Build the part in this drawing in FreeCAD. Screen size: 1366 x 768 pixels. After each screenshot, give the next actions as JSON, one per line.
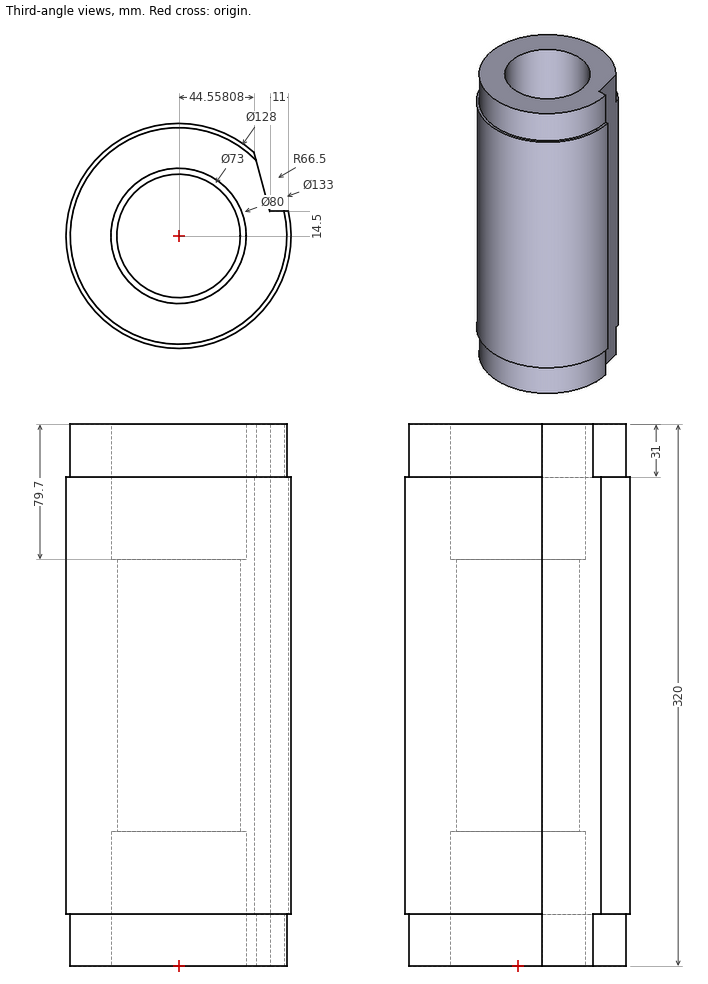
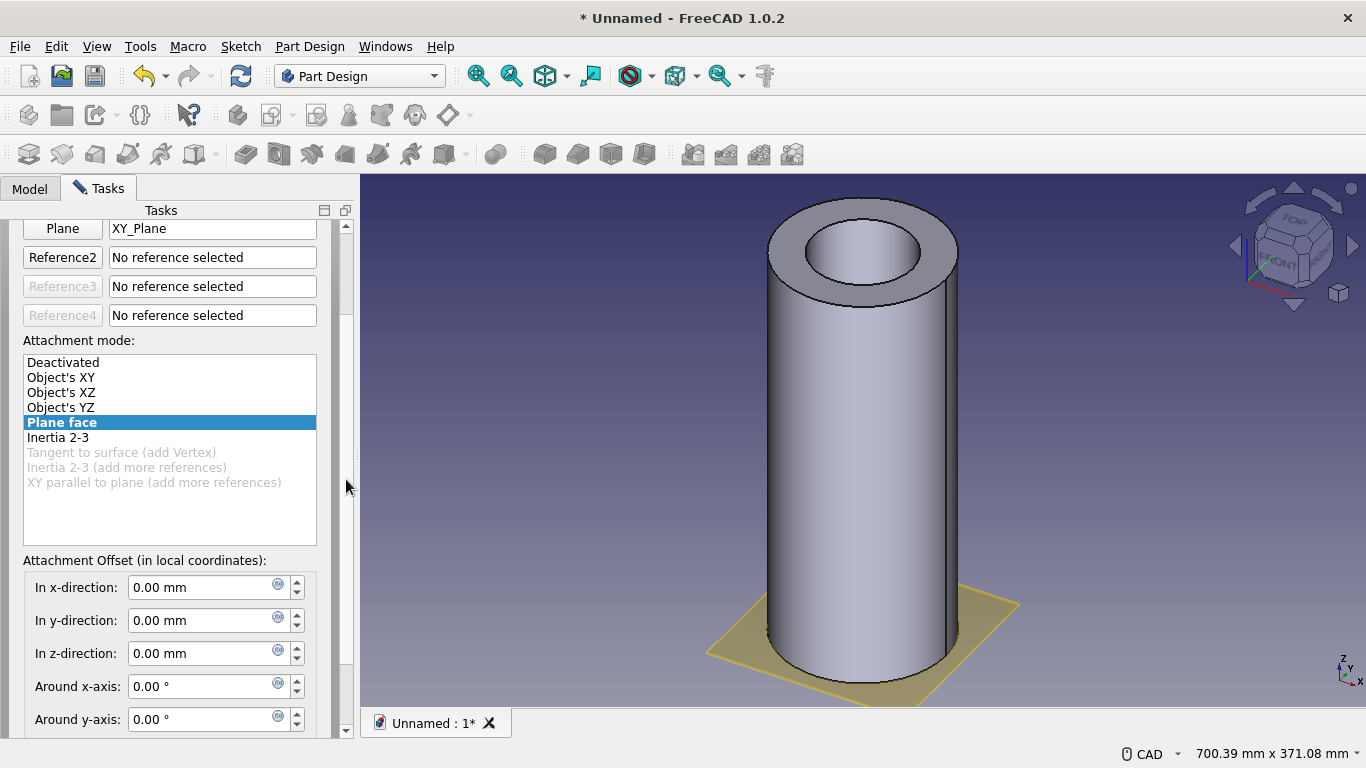
{"action": "triple_click", "coordinate": [210, 654]}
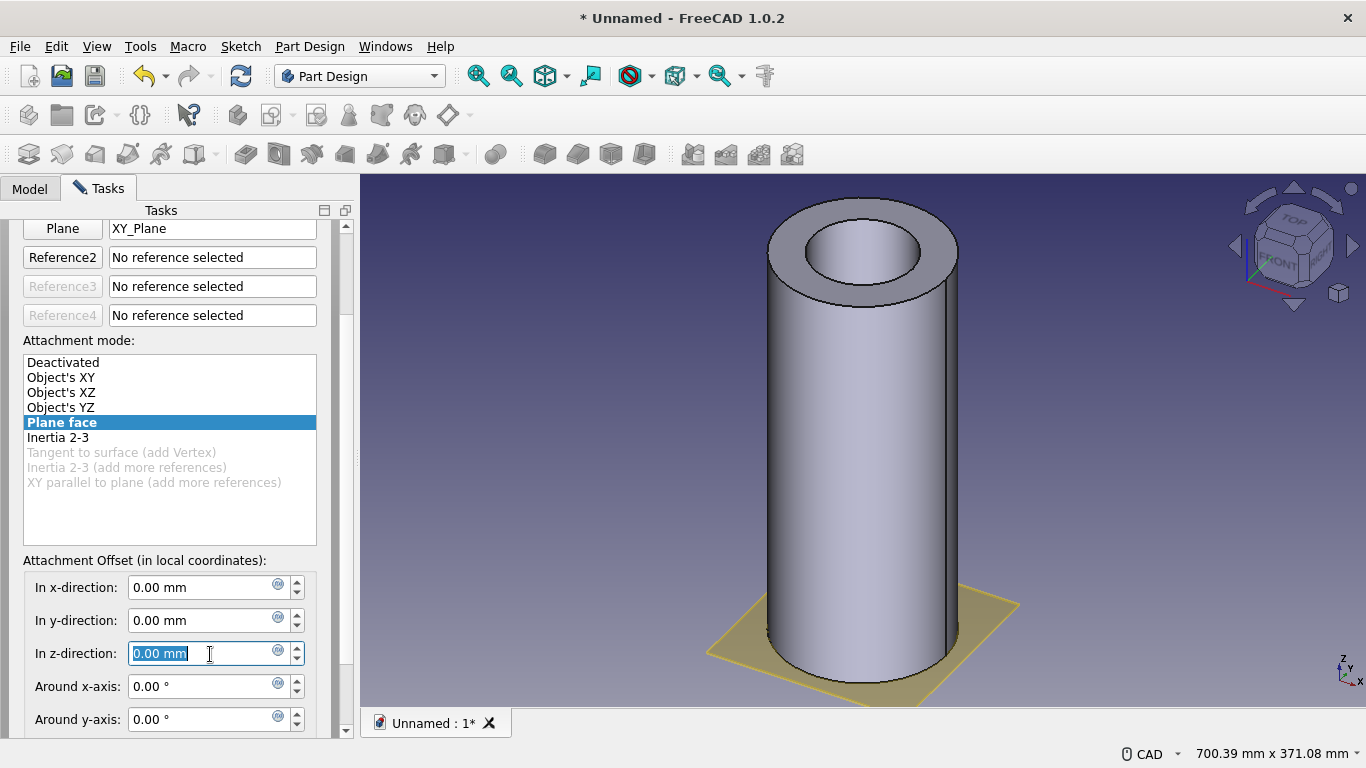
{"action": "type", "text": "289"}
{"action": "key", "text": "Tab"}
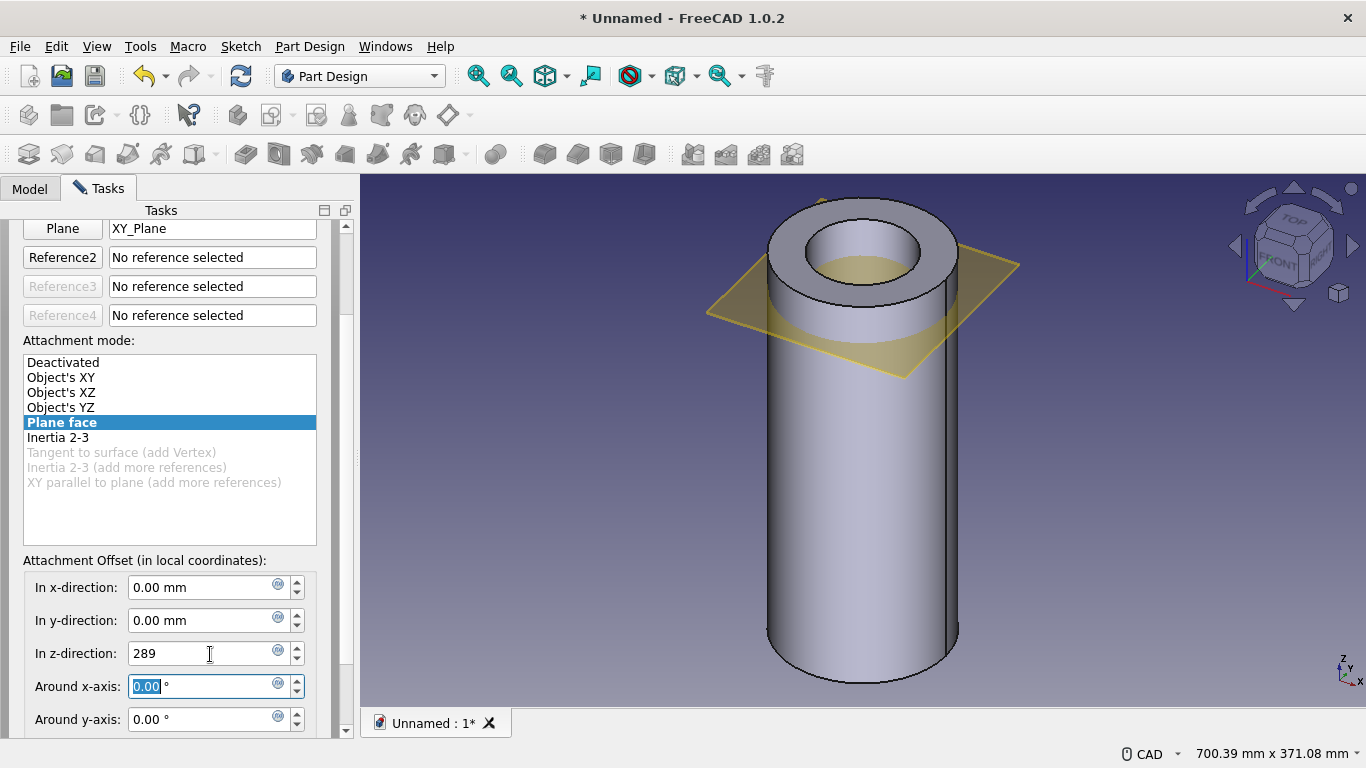
{"action": "scroll", "coordinate": [346, 479], "scroll_direction": "up", "scroll_amount": 3}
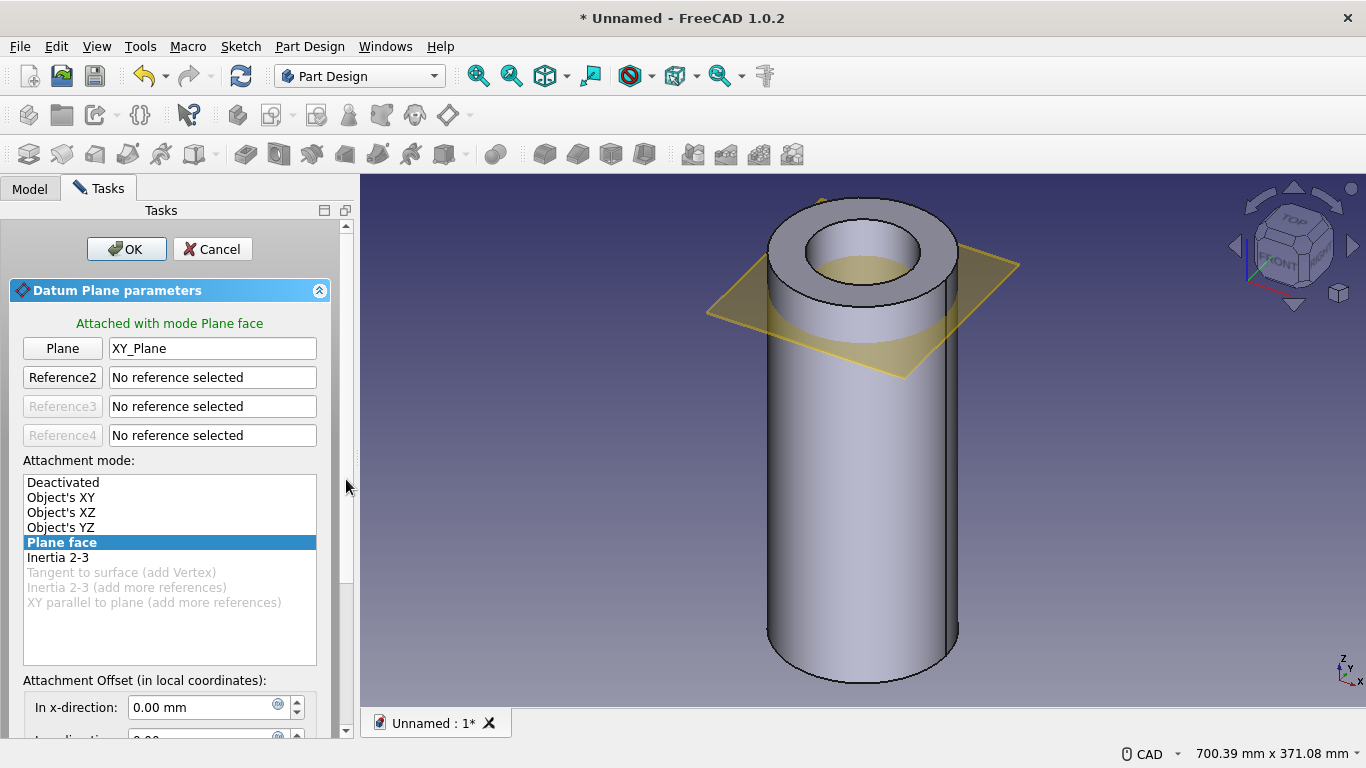
{"action": "left_click", "coordinate": [127, 249]}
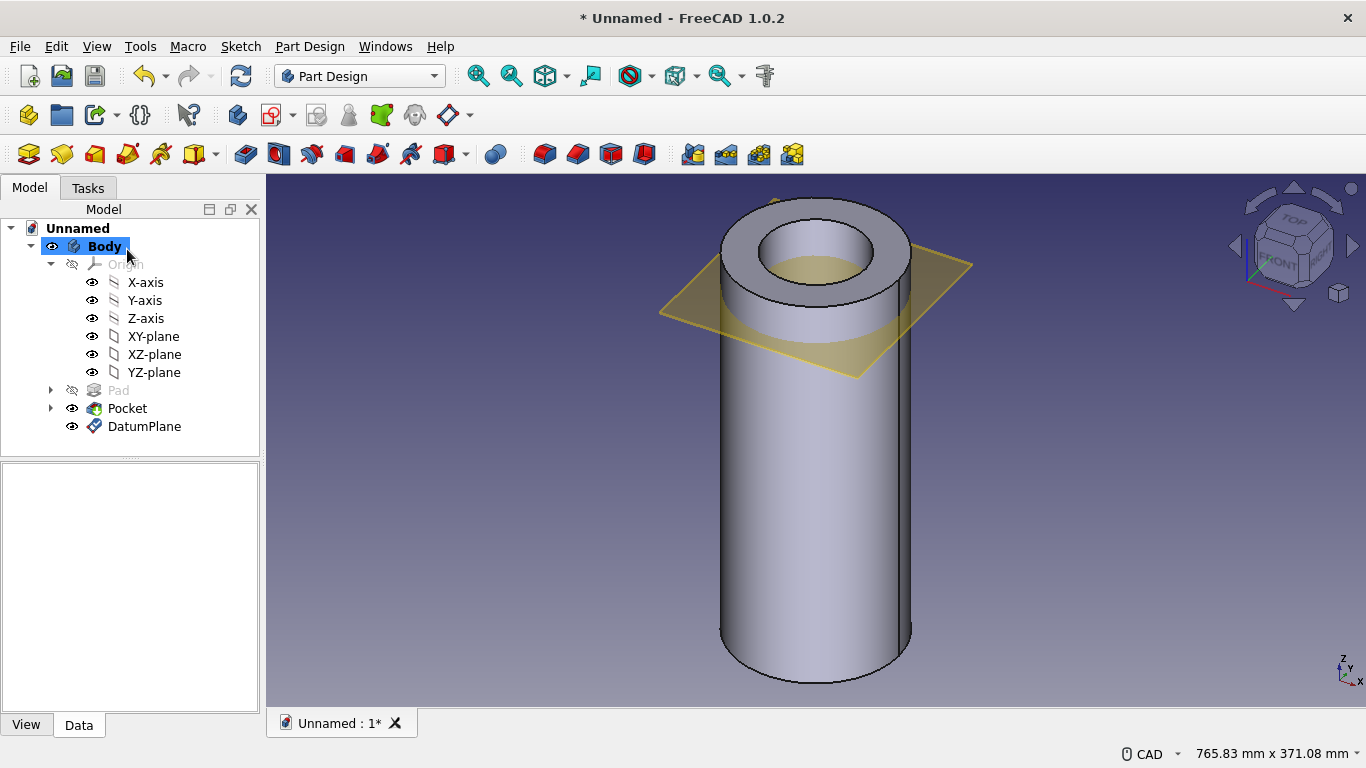
{"action": "left_click", "coordinate": [117, 426]}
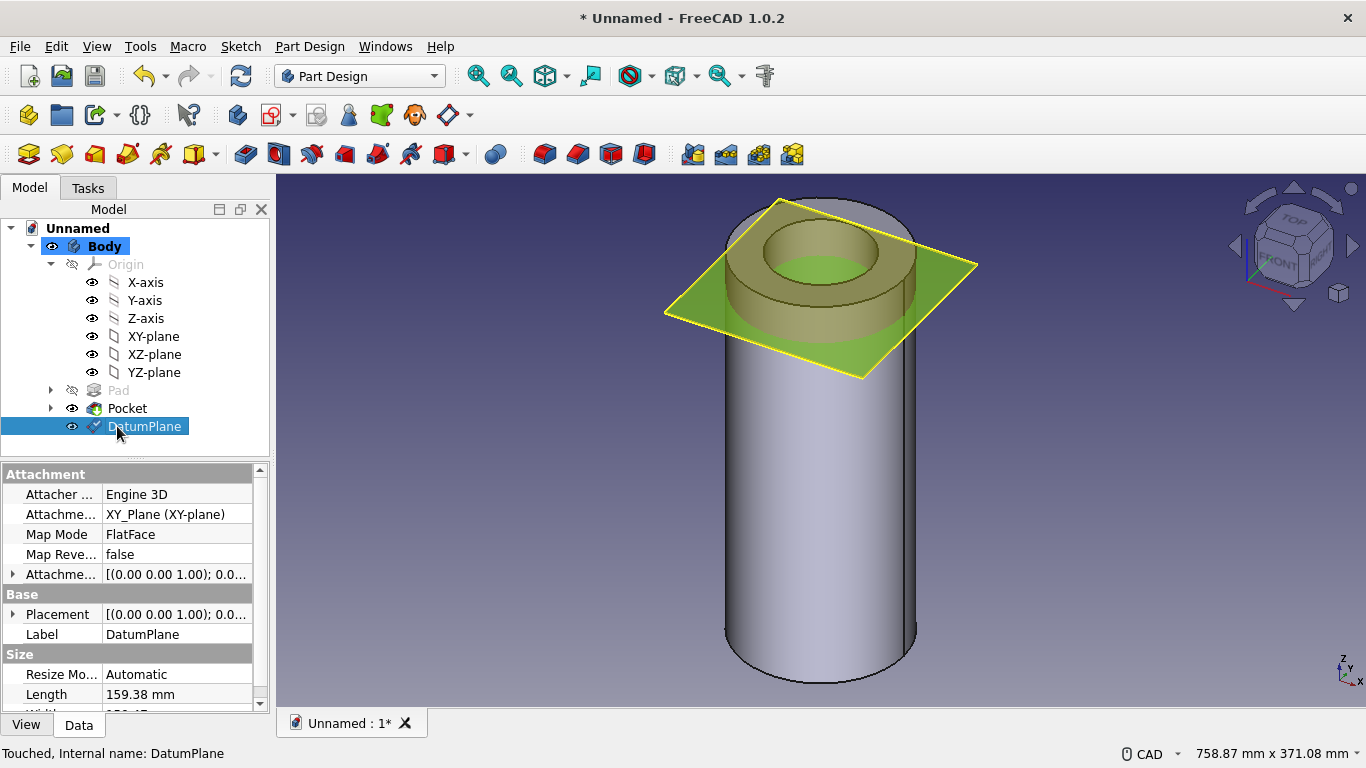
{"action": "left_click", "coordinate": [270, 116]}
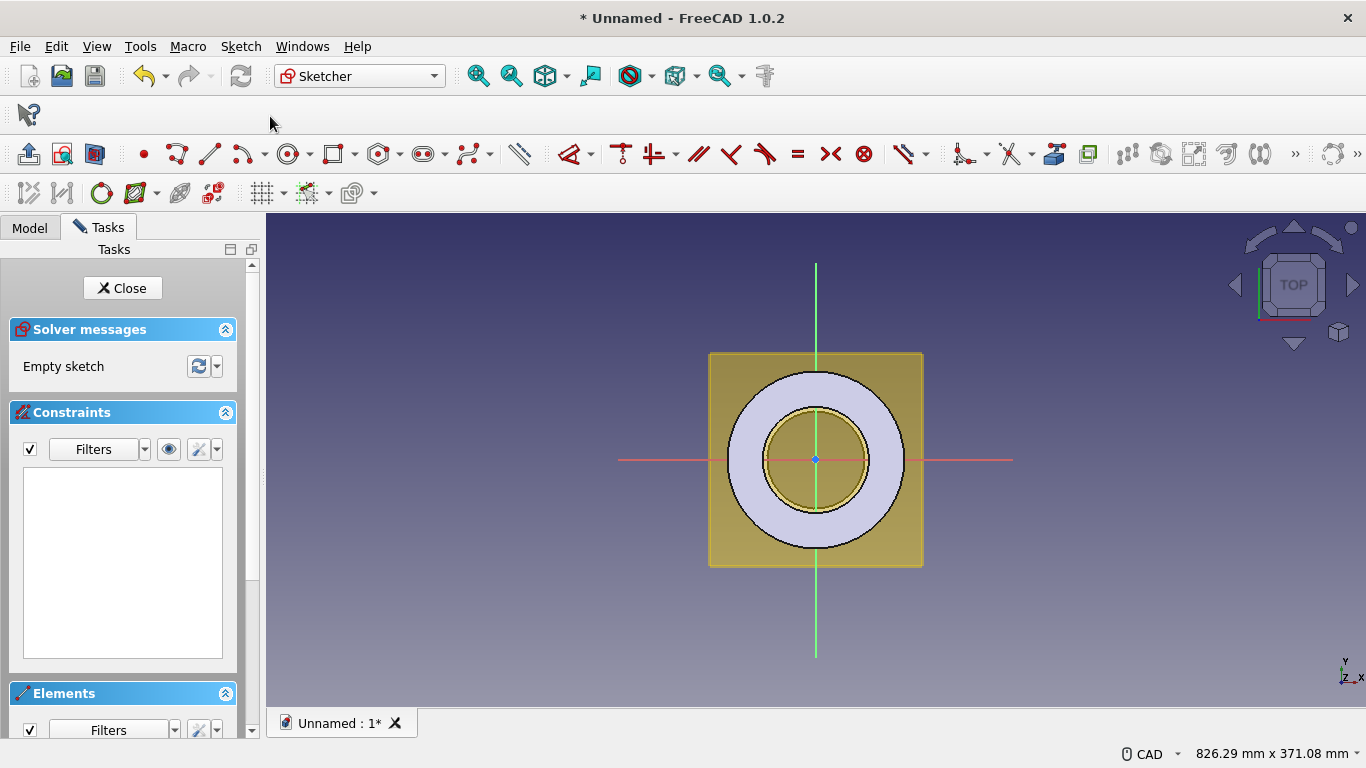
{"action": "left_click", "coordinate": [95, 154]}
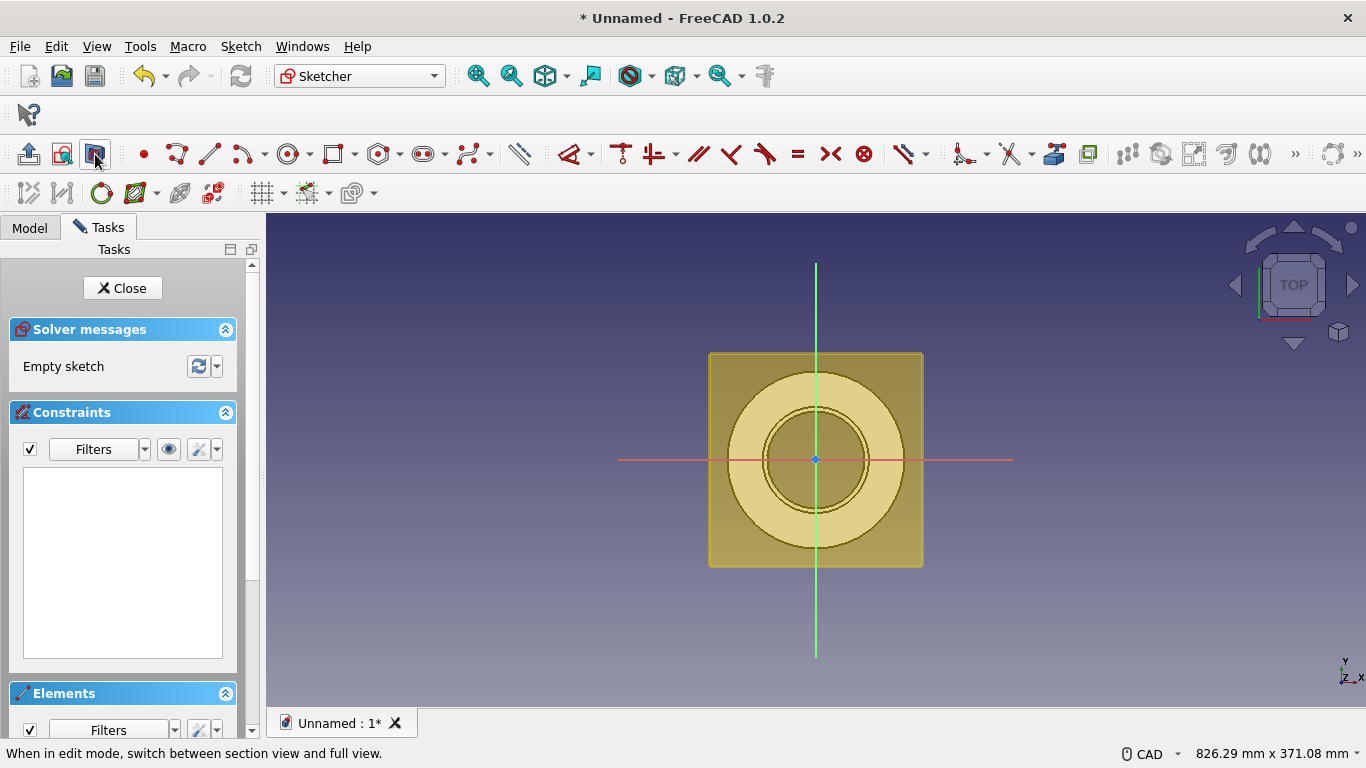
{"action": "scroll", "coordinate": [899, 460], "scroll_direction": "up", "scroll_amount": 3}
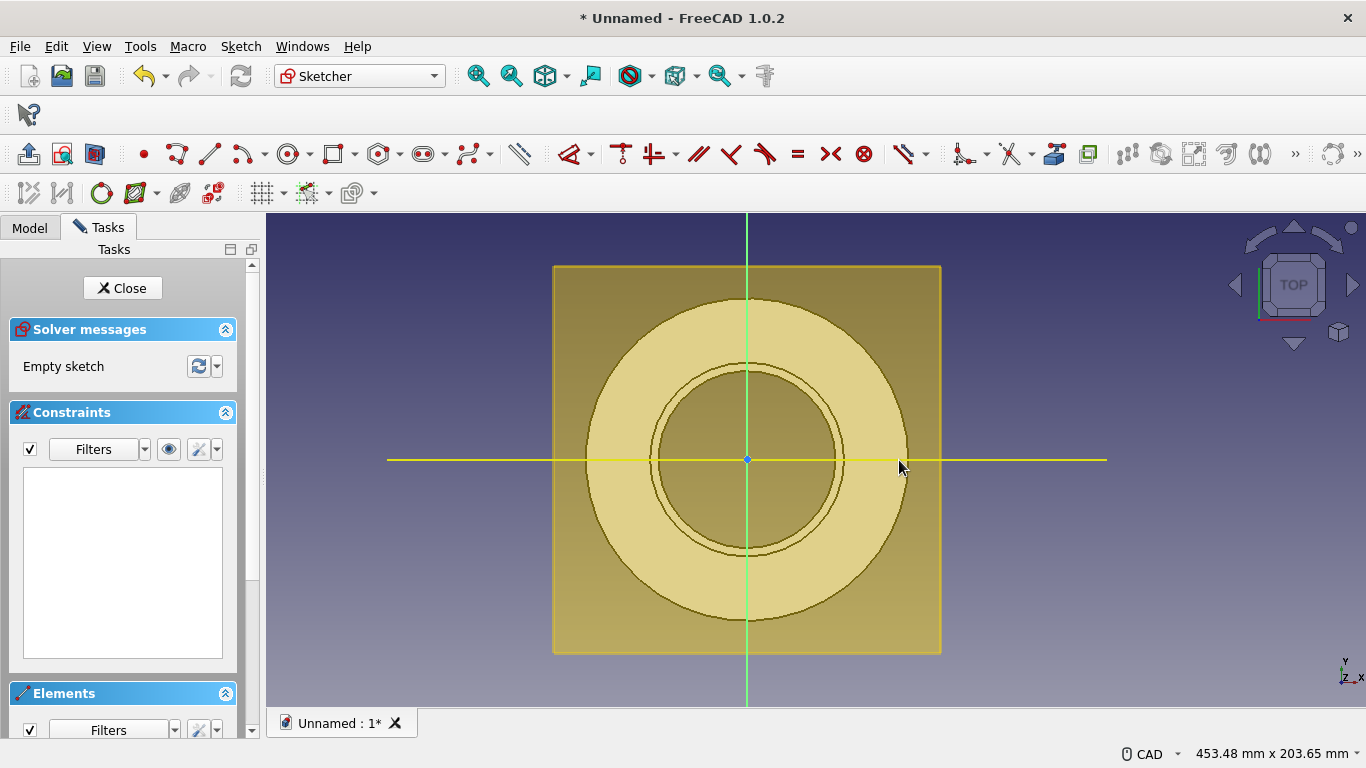
{"action": "left_click", "coordinate": [288, 154]}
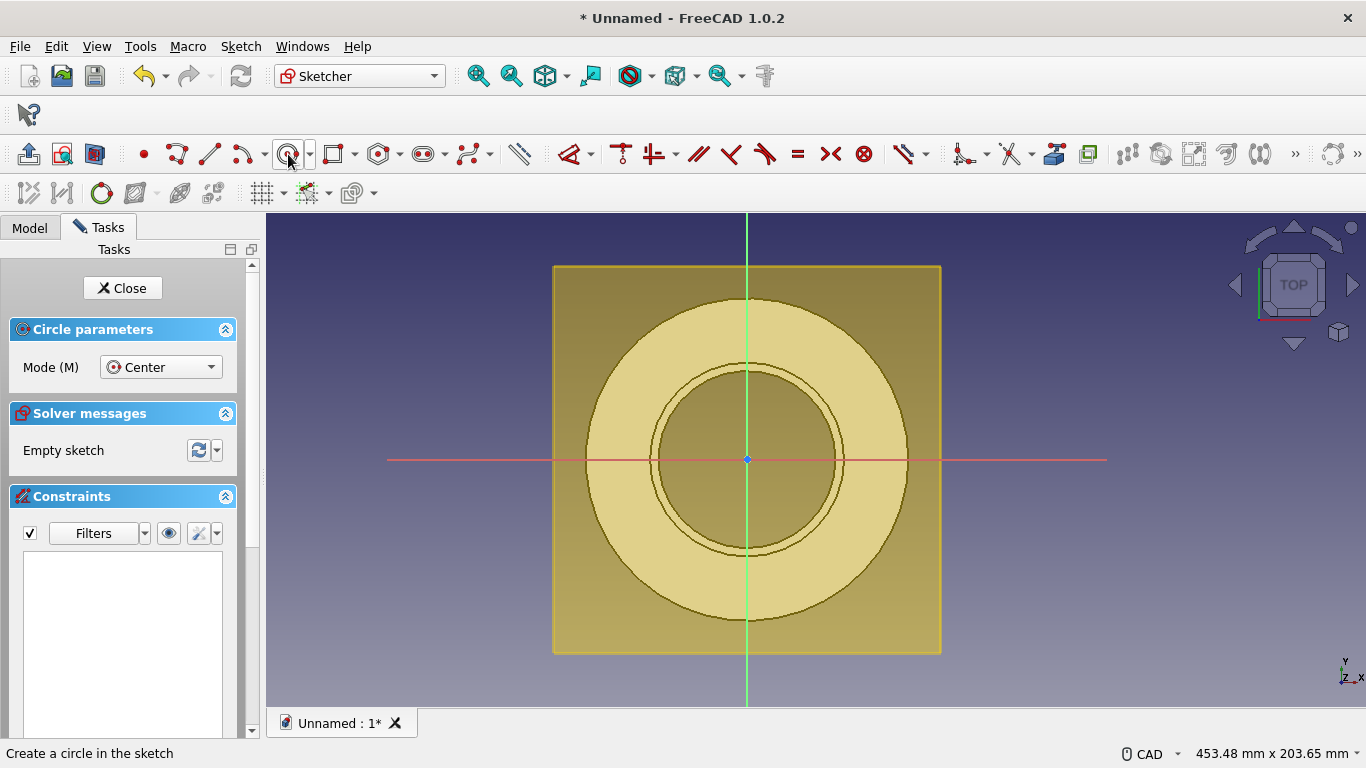
{"action": "left_click", "coordinate": [747, 460]}
{"action": "mouse_move", "coordinate": [861, 346]}